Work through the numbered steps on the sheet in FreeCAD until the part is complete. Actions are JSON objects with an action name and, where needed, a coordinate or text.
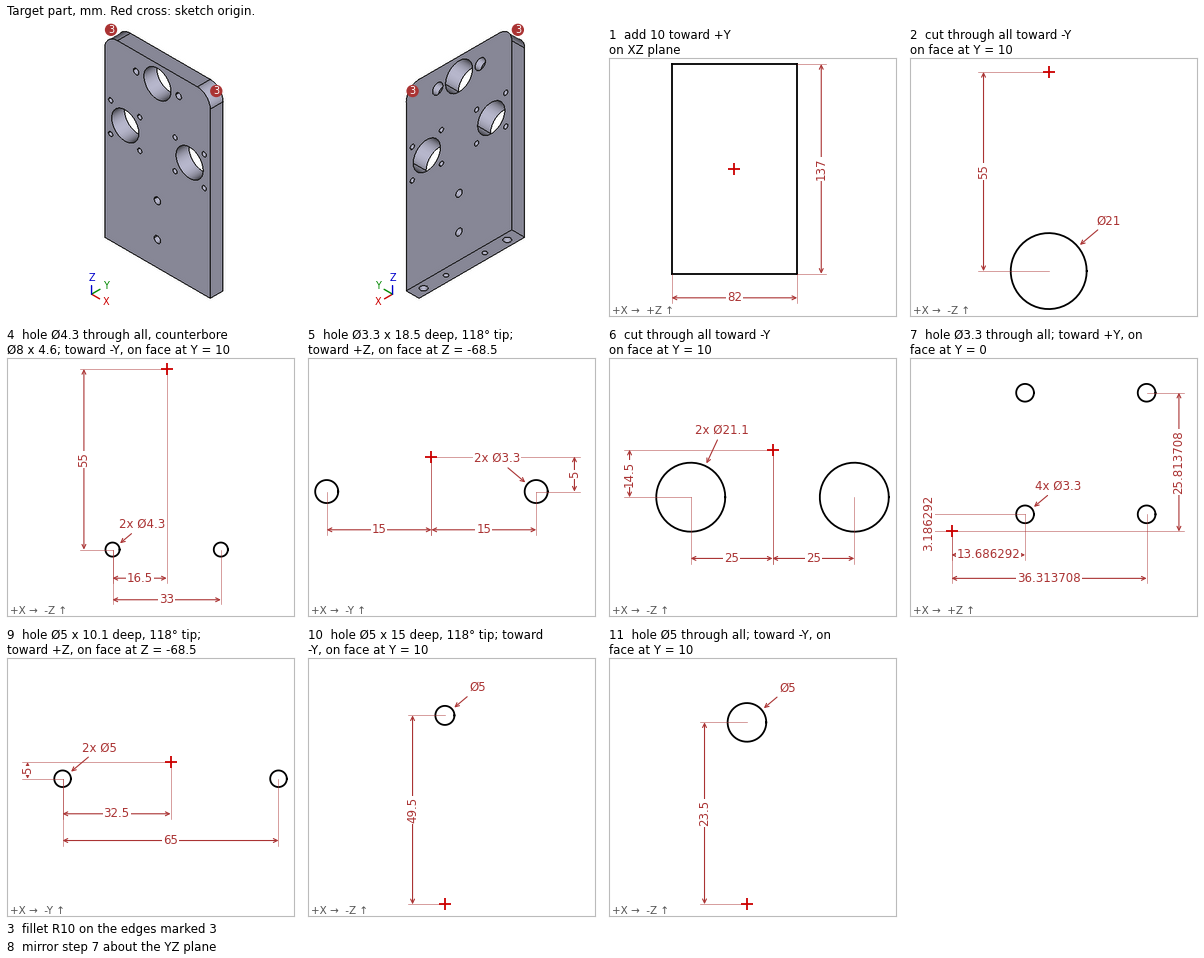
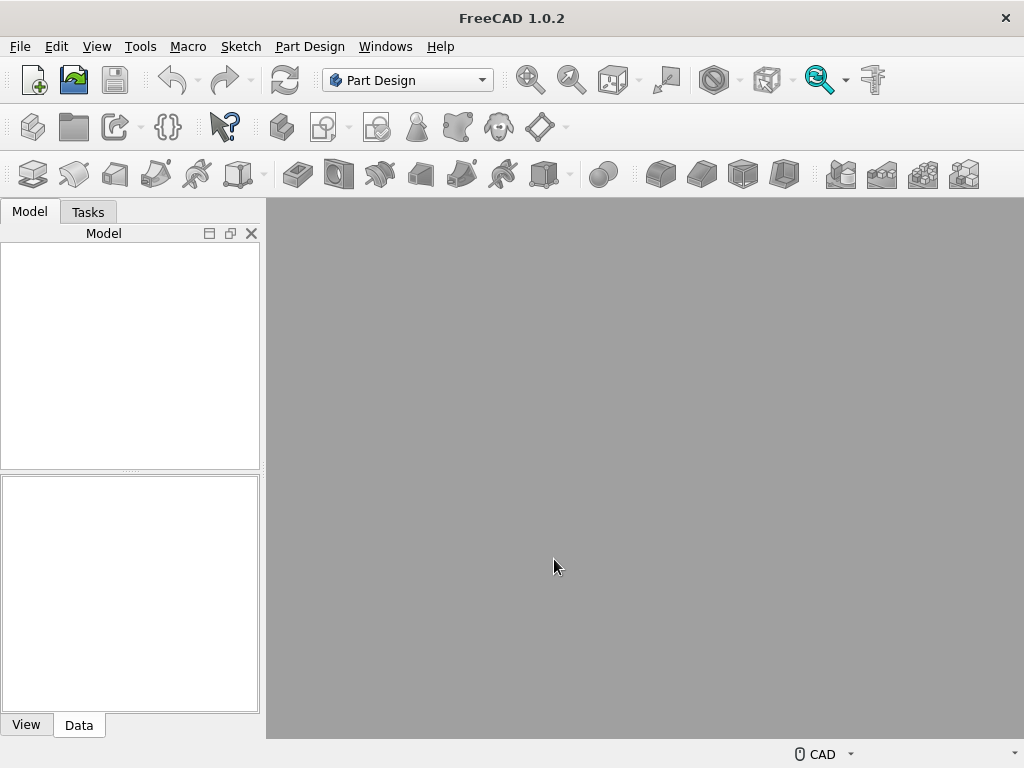
{"action": "key", "text": "ctrl+n"}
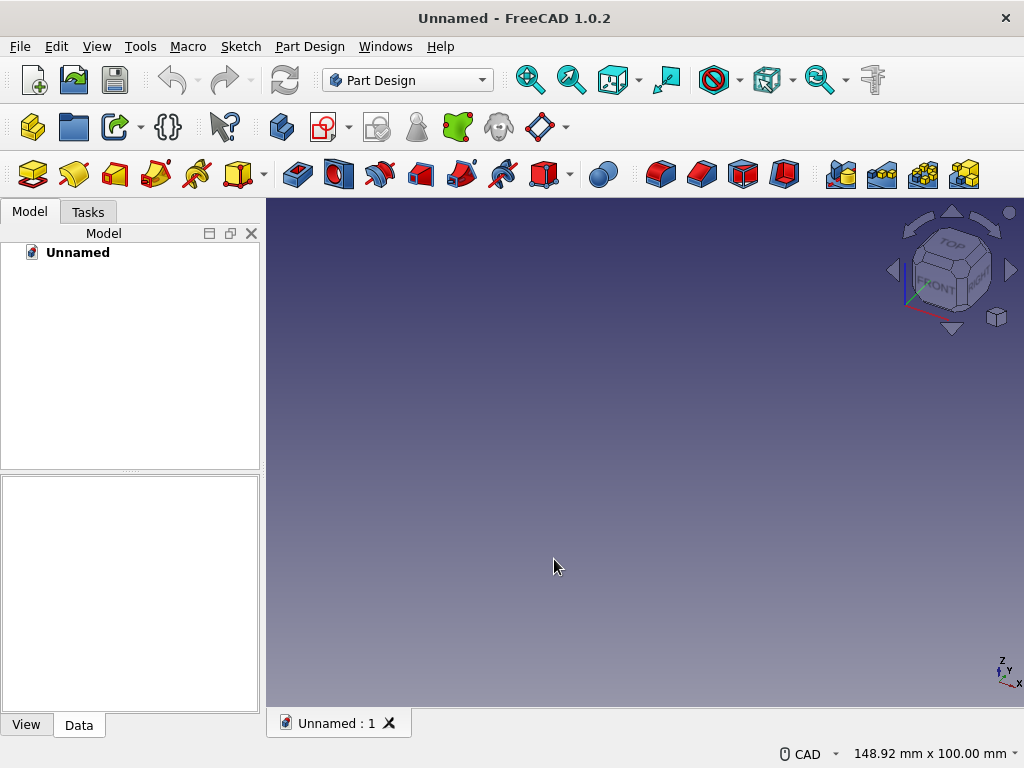
{"action": "left_click", "coordinate": [322, 128]}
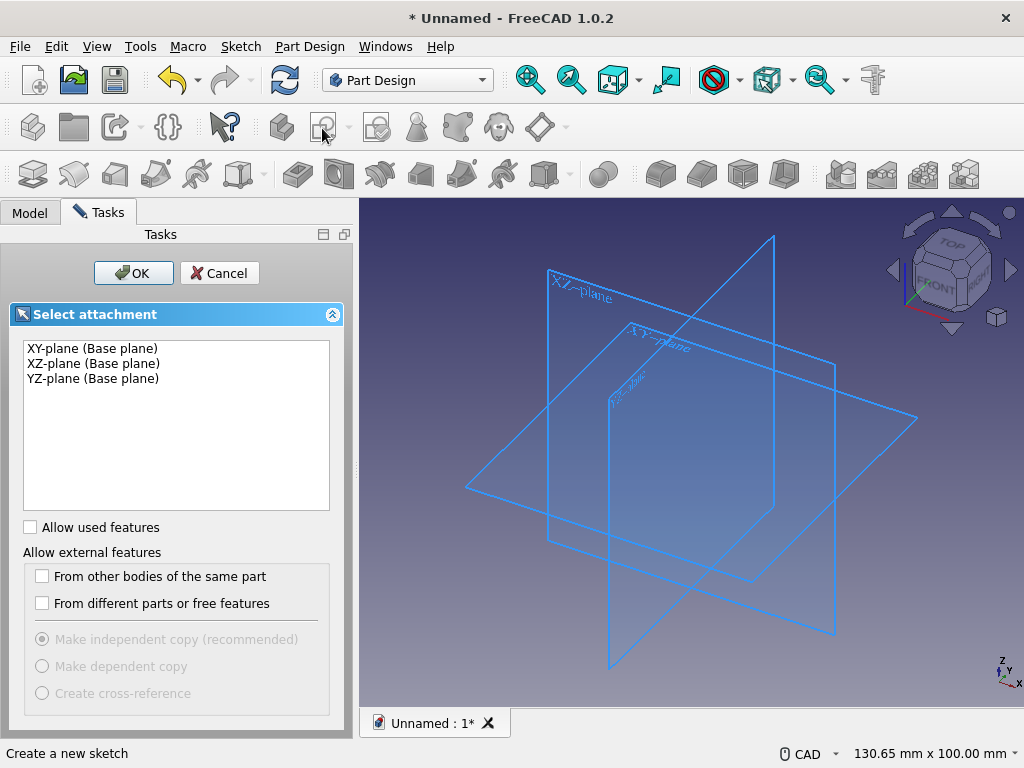
{"action": "left_click", "coordinate": [84, 364]}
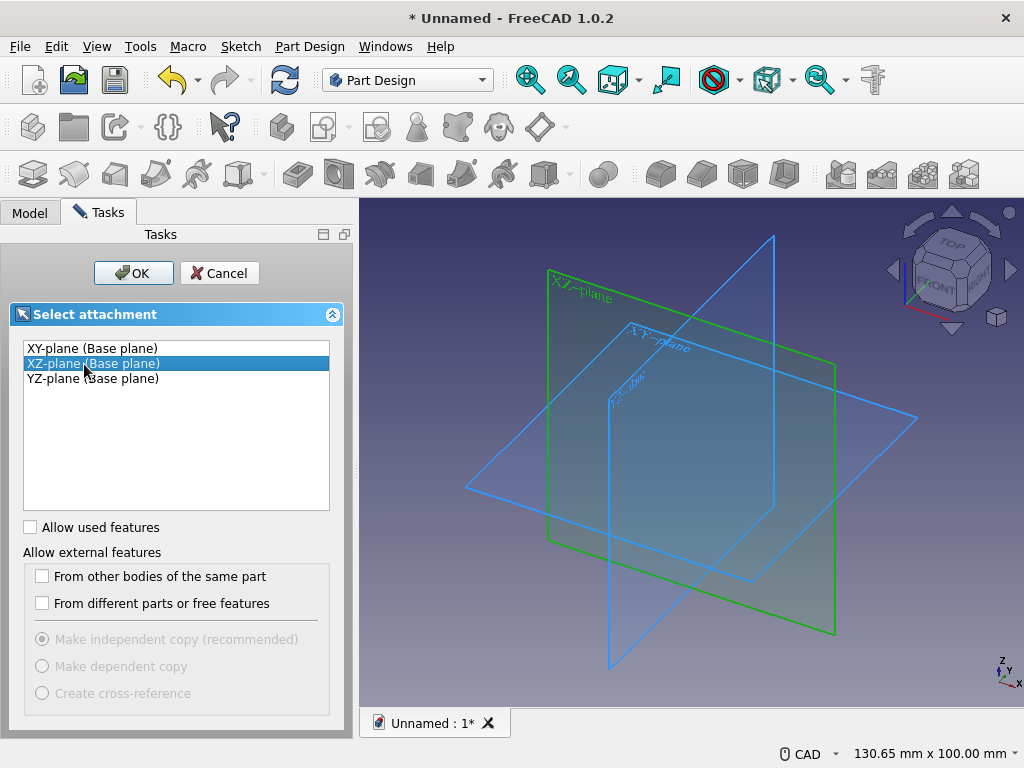
{"action": "left_click", "coordinate": [134, 273]}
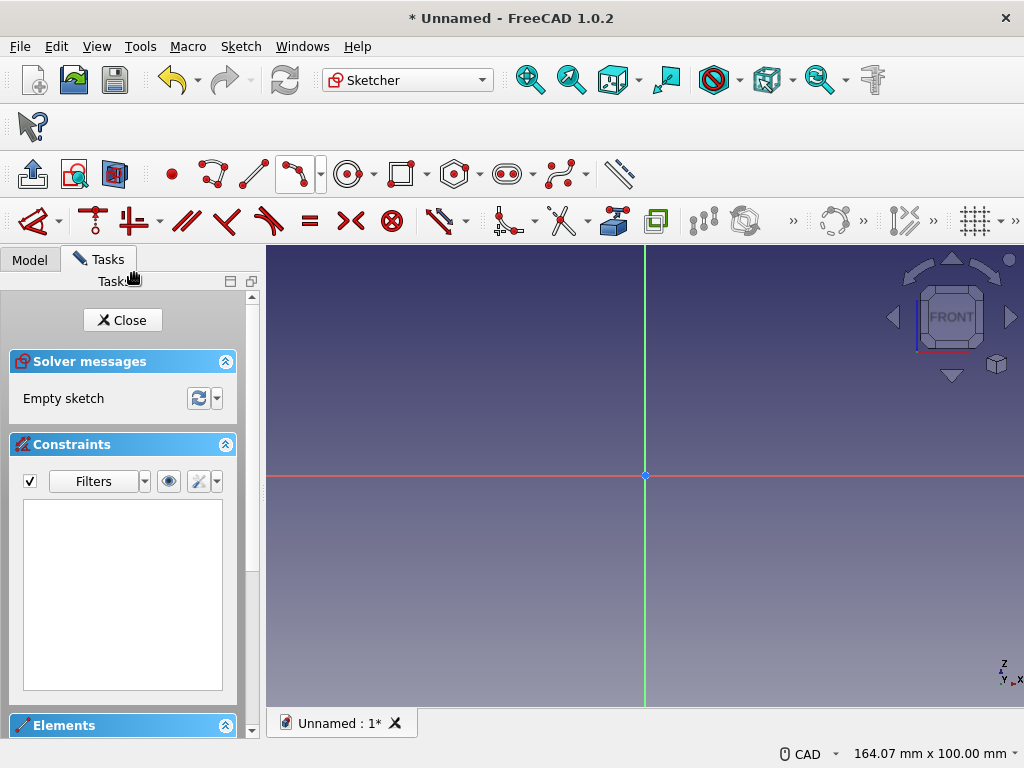
{"action": "scroll", "coordinate": [521, 476], "scroll_direction": "down", "scroll_amount": 4}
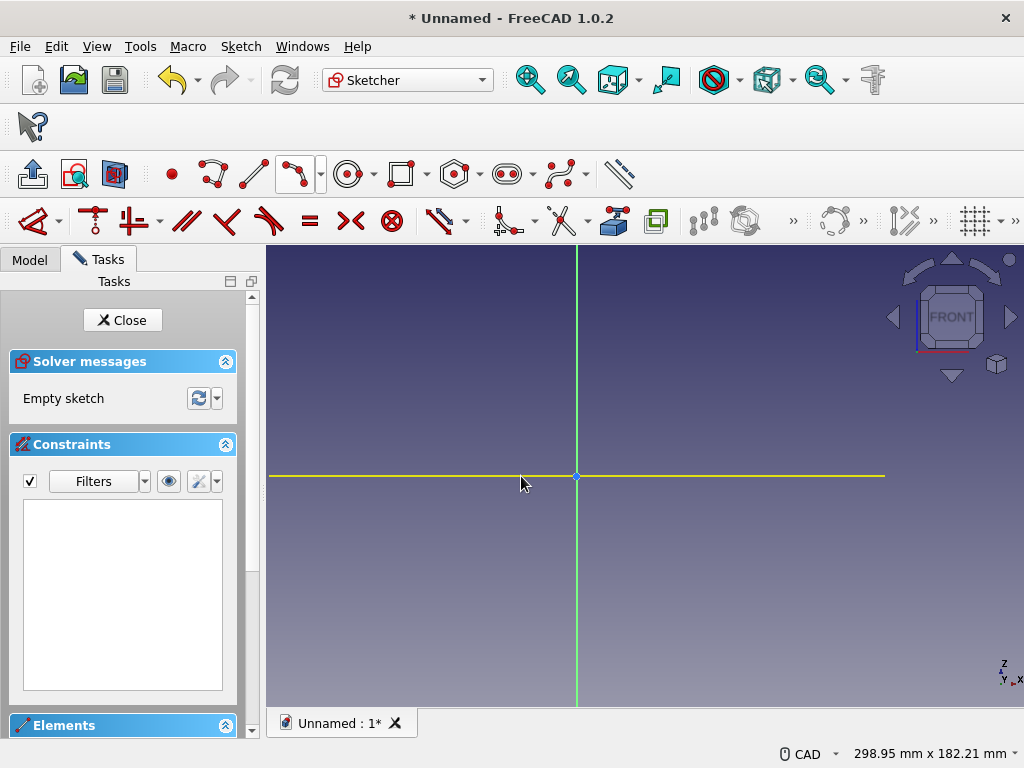
{"action": "key", "text": "g v"}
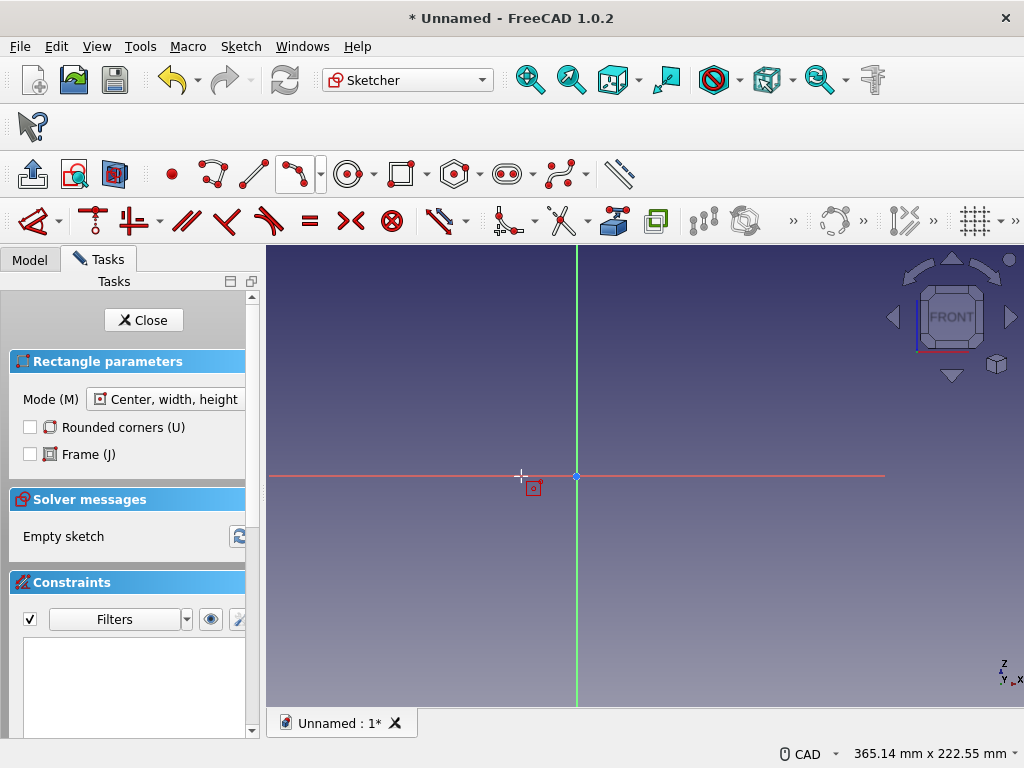
{"action": "left_click", "coordinate": [577, 476]}
{"action": "mouse_move", "coordinate": [662, 334]}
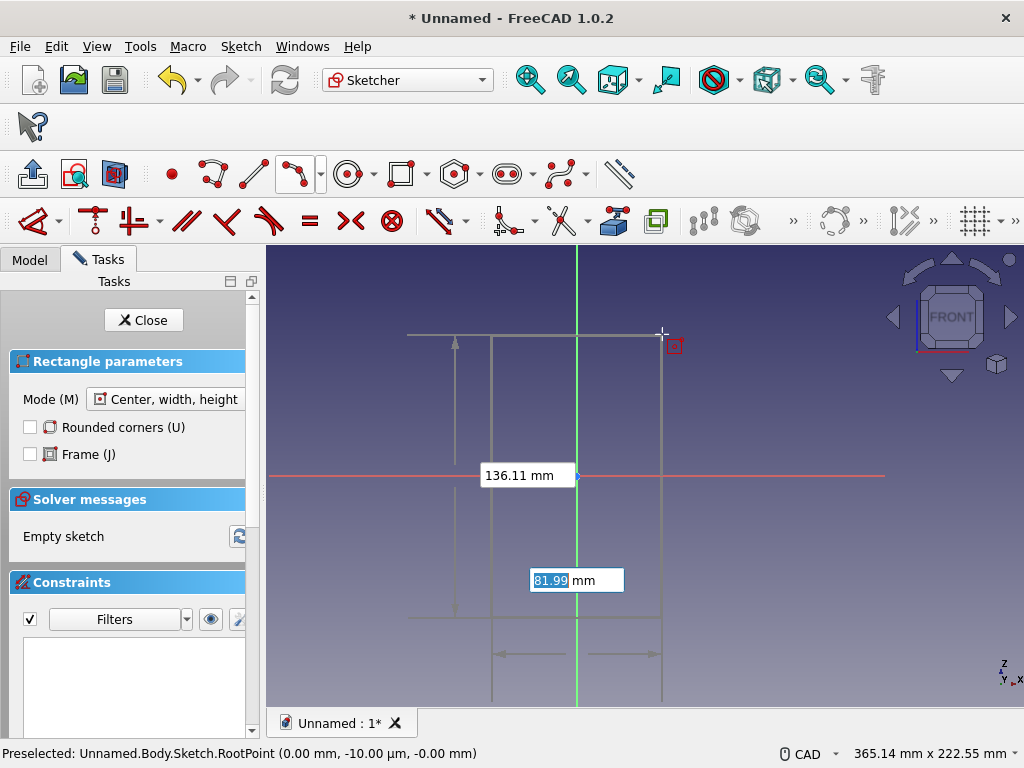
{"action": "type", "text": "82"}
{"action": "key", "text": "Tab"}
{"action": "type", "text": "137"}
{"action": "key", "text": "Return"}
{"action": "key", "text": "Escape"}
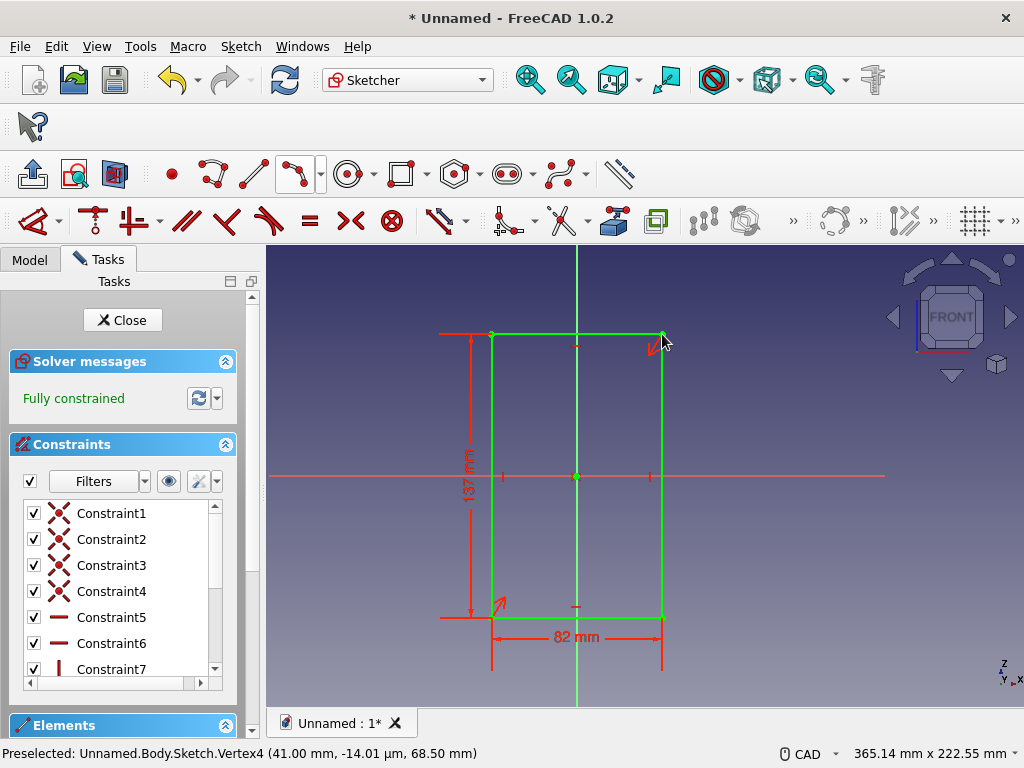
{"action": "left_click", "coordinate": [123, 320]}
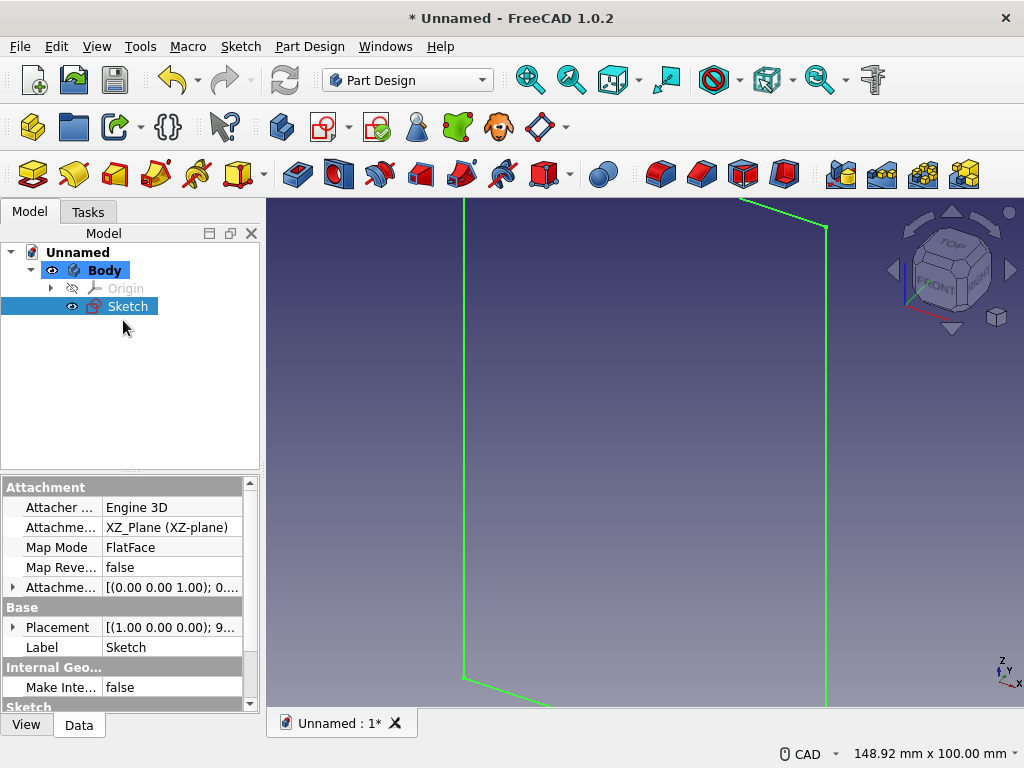
{"action": "left_click", "coordinate": [33, 174]}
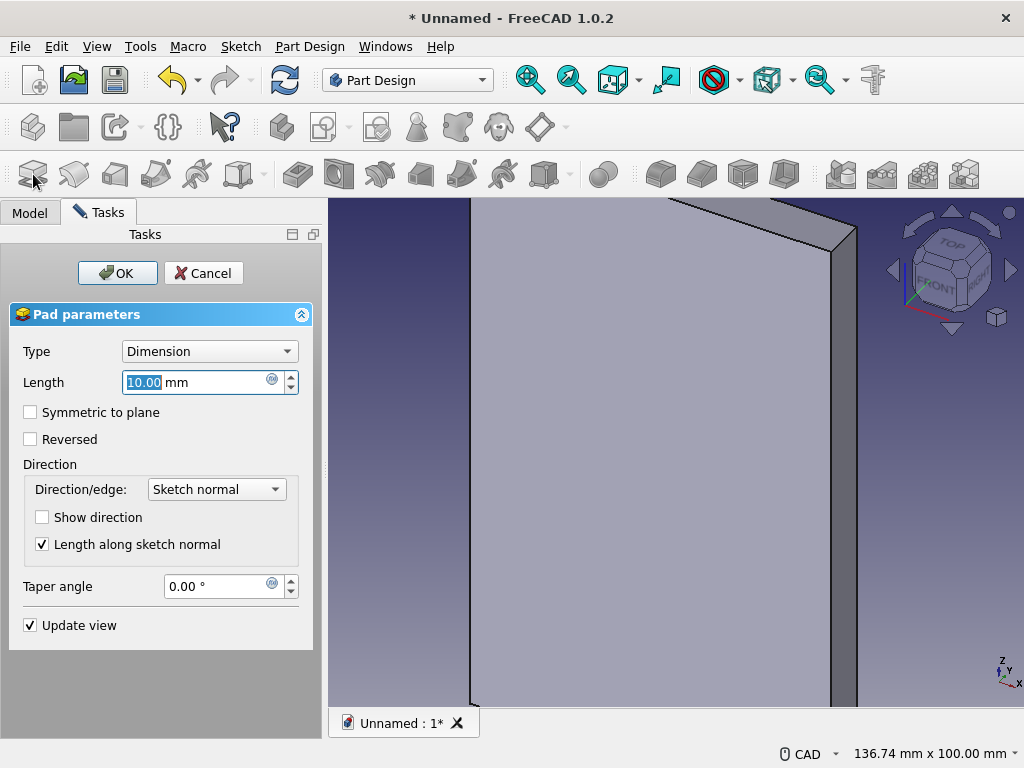
{"action": "type", "text": "10"}
{"action": "key", "text": "Tab"}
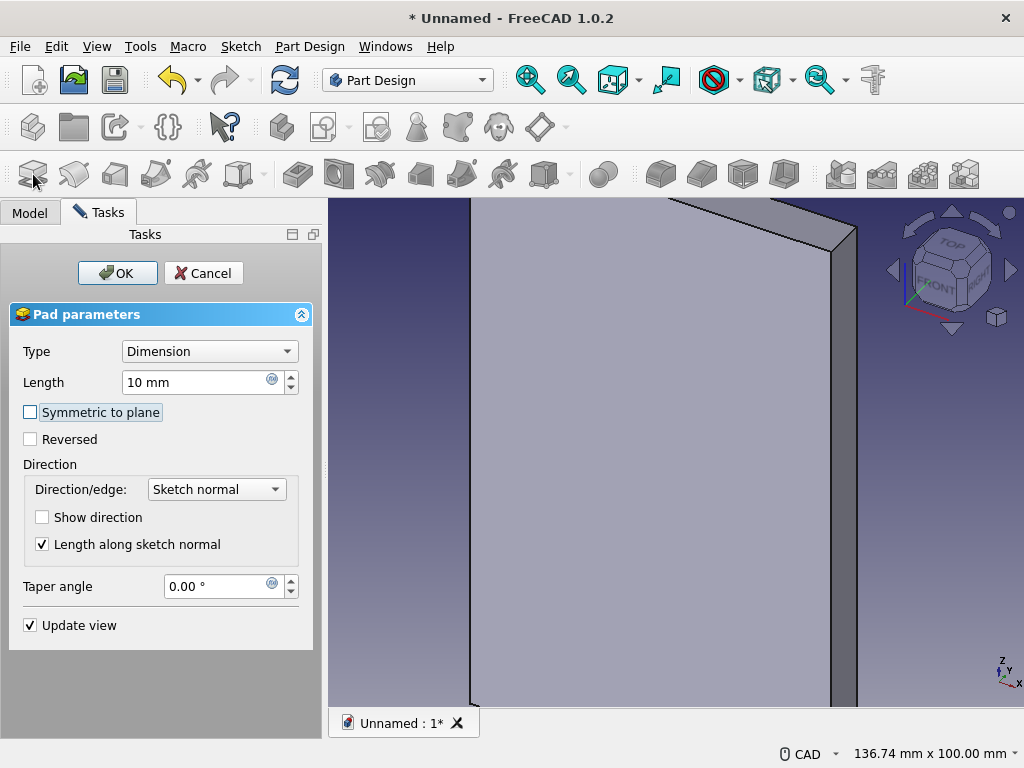
{"action": "left_click", "coordinate": [31, 439]}